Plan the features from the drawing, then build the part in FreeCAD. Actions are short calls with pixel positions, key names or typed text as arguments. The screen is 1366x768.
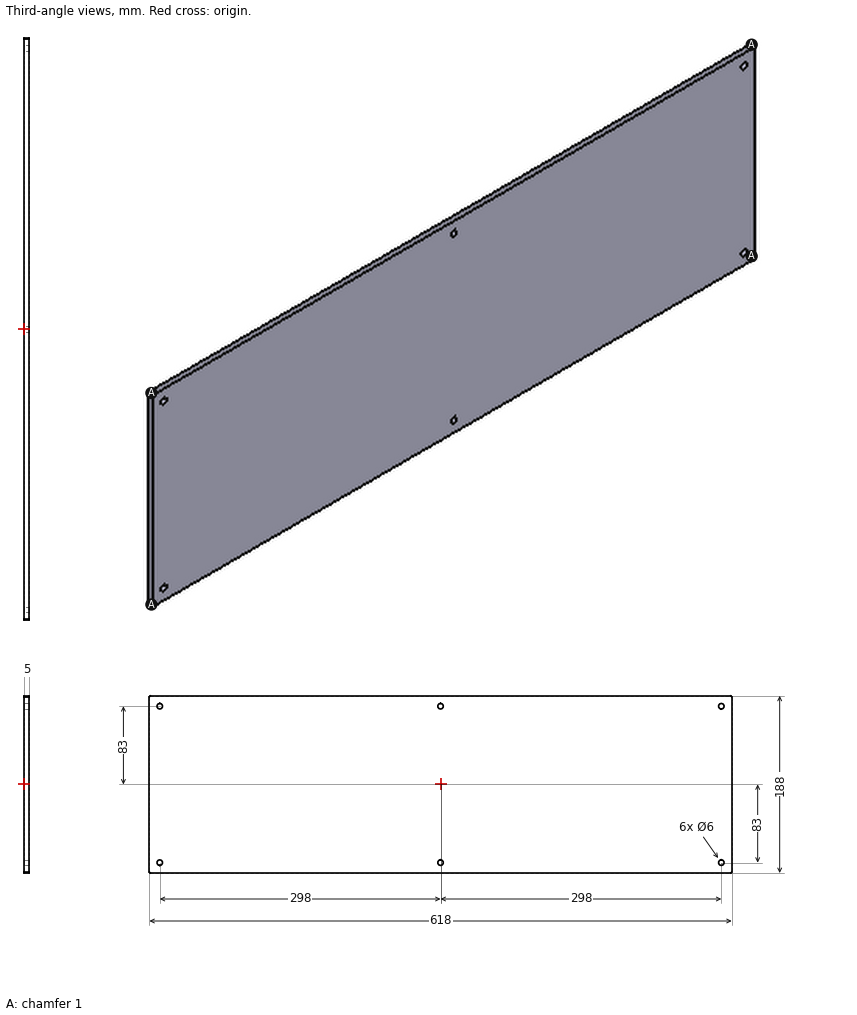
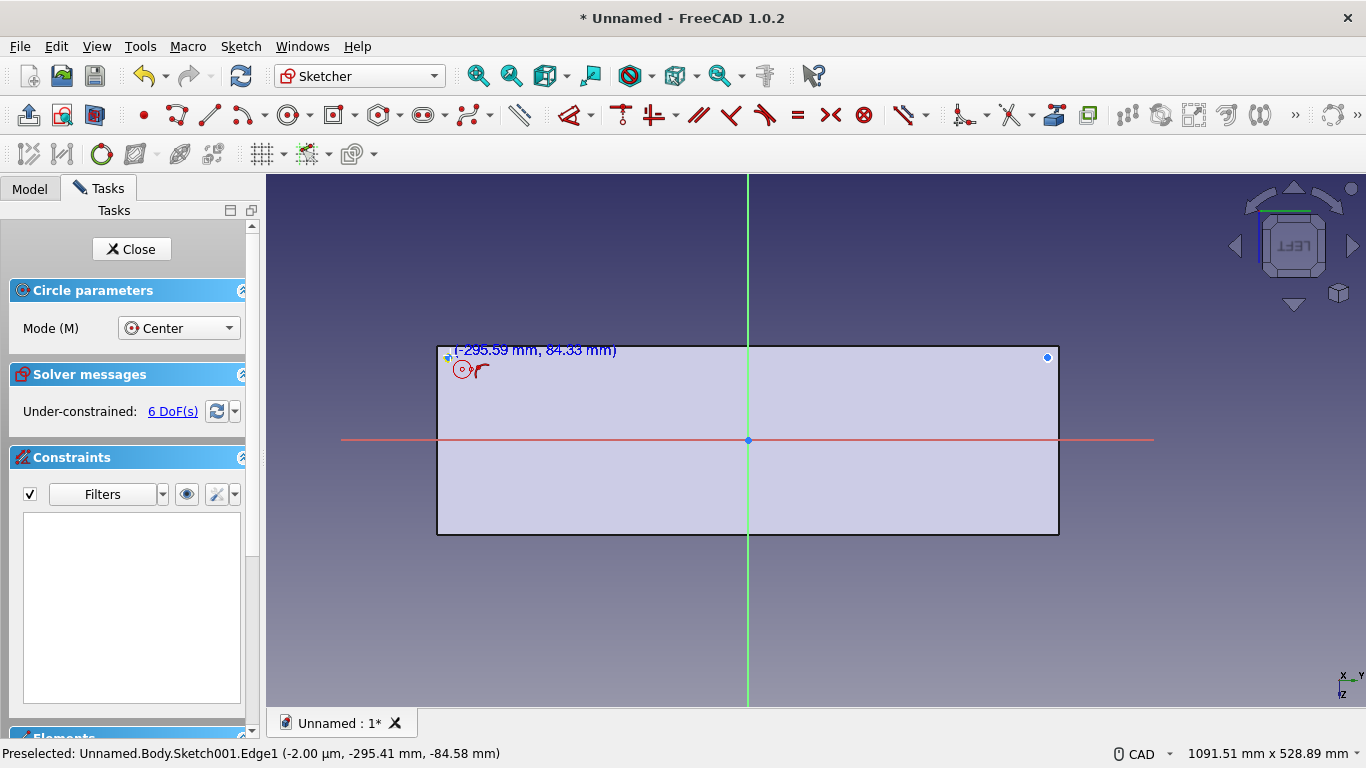
scroll(448, 524, up, 11)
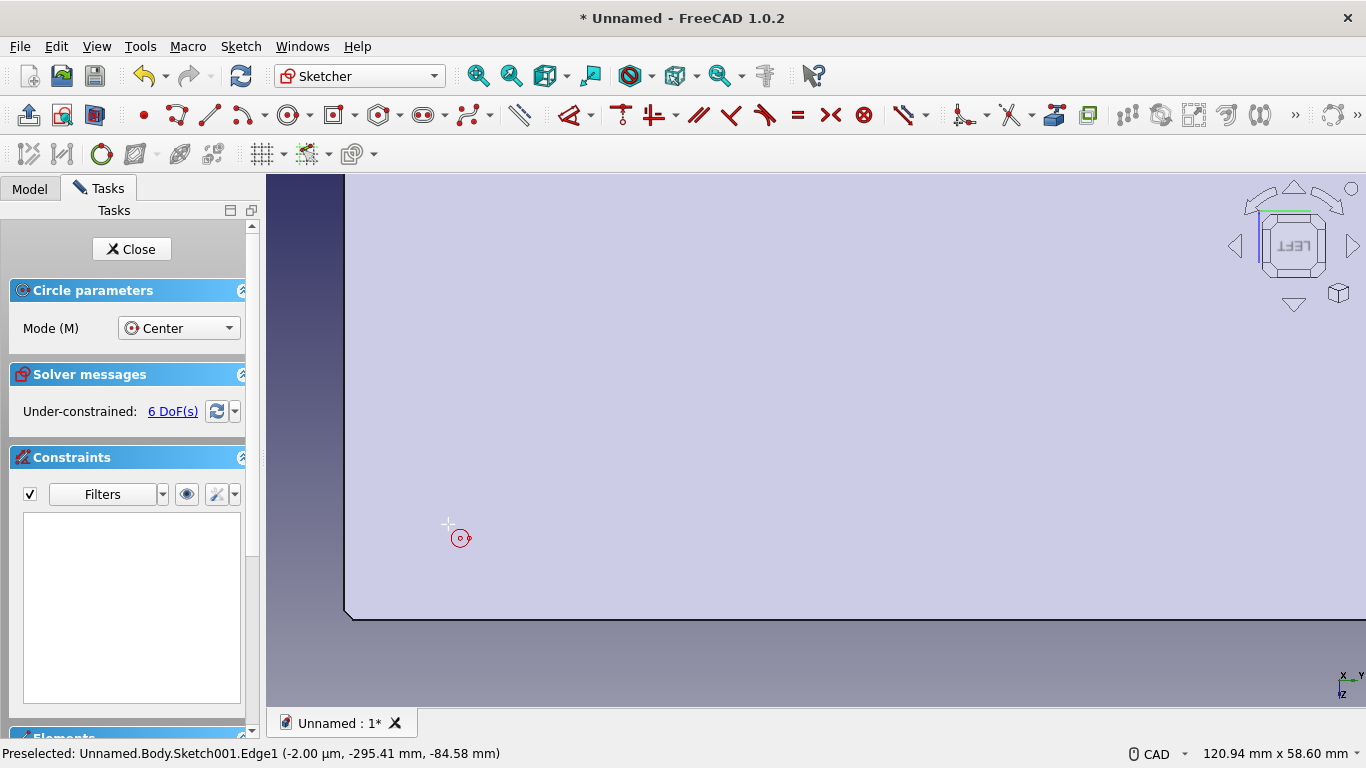
scroll(448, 525, down, 11)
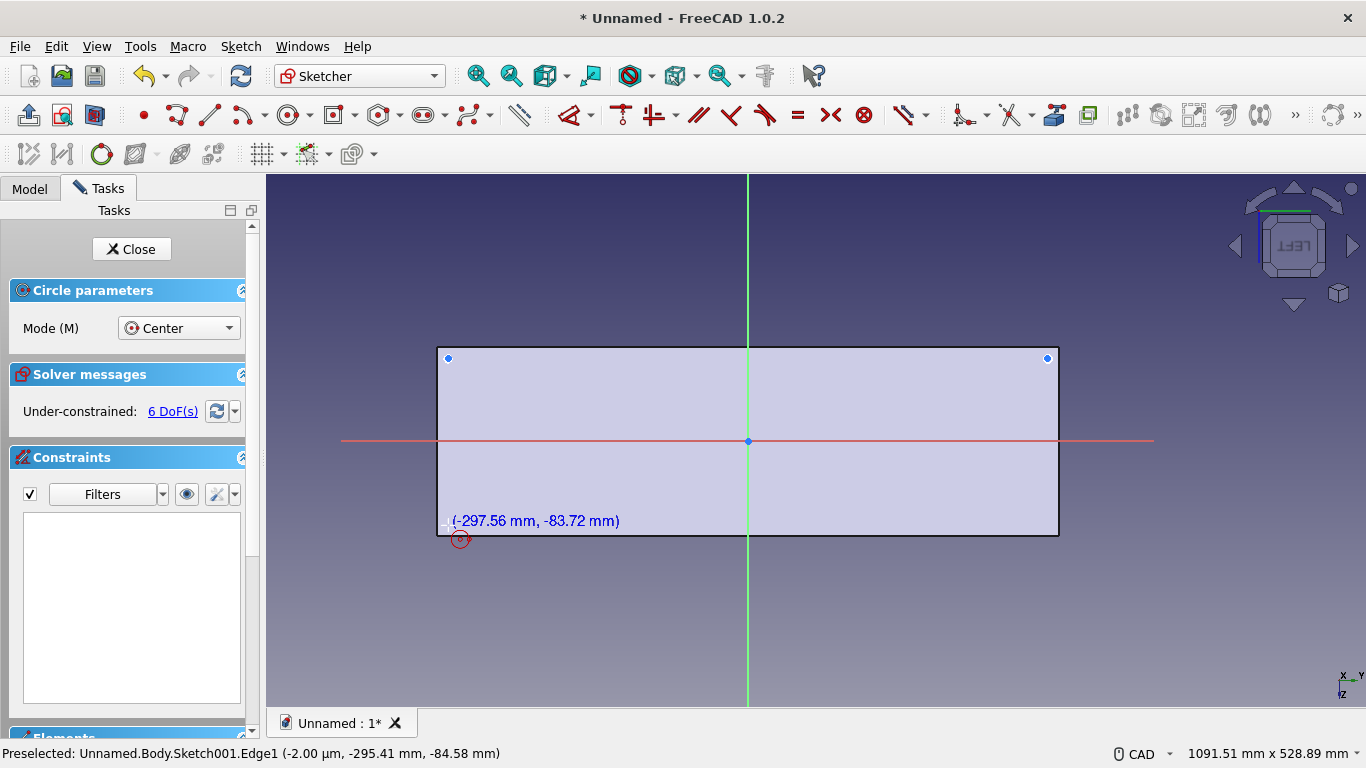
click(448, 525)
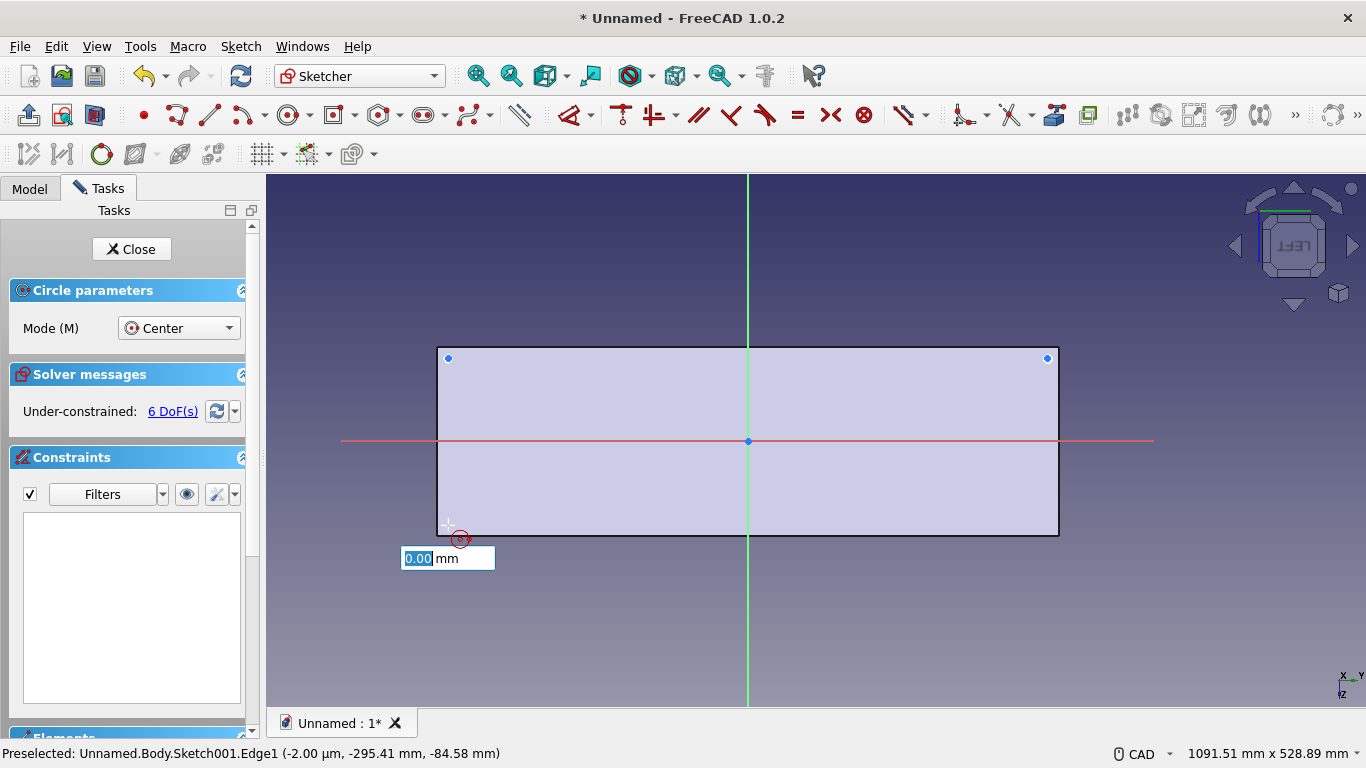
scroll(450, 523, up, 9)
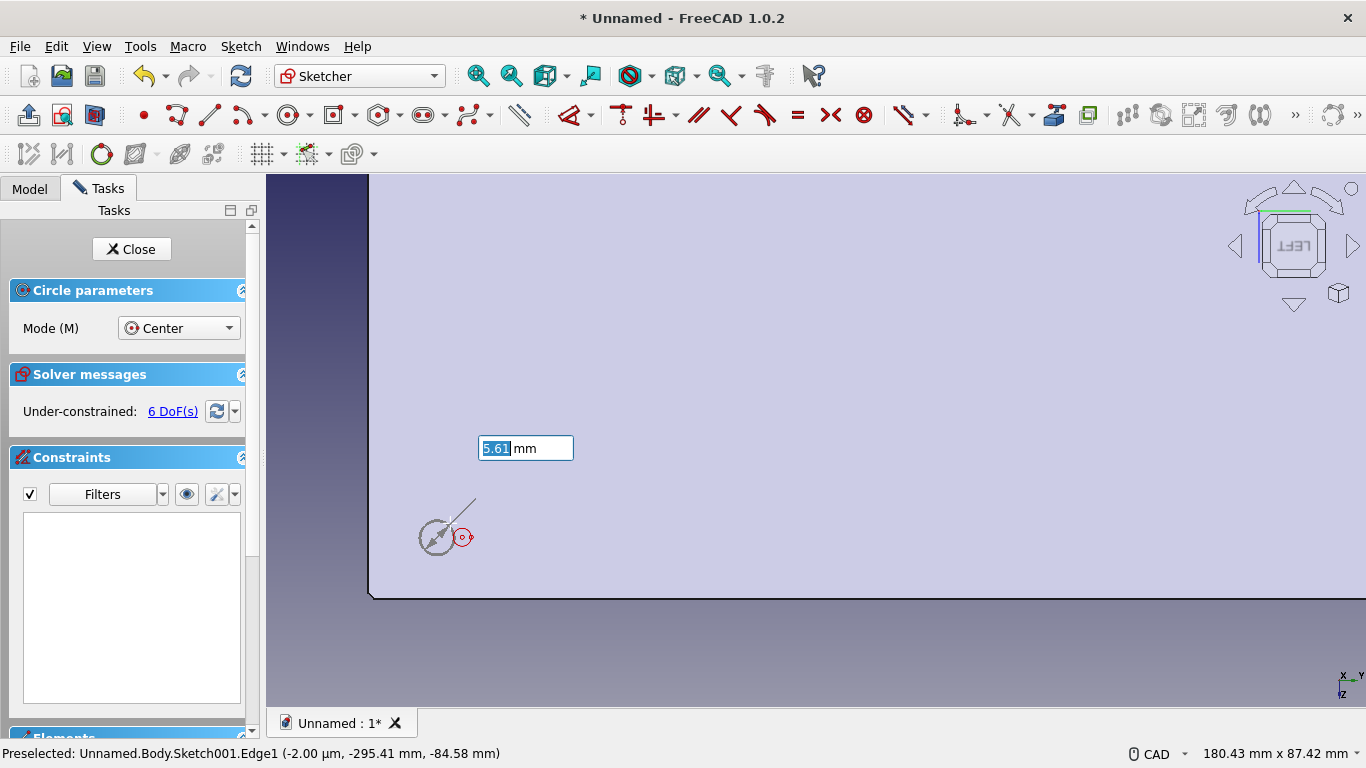
click(448, 519)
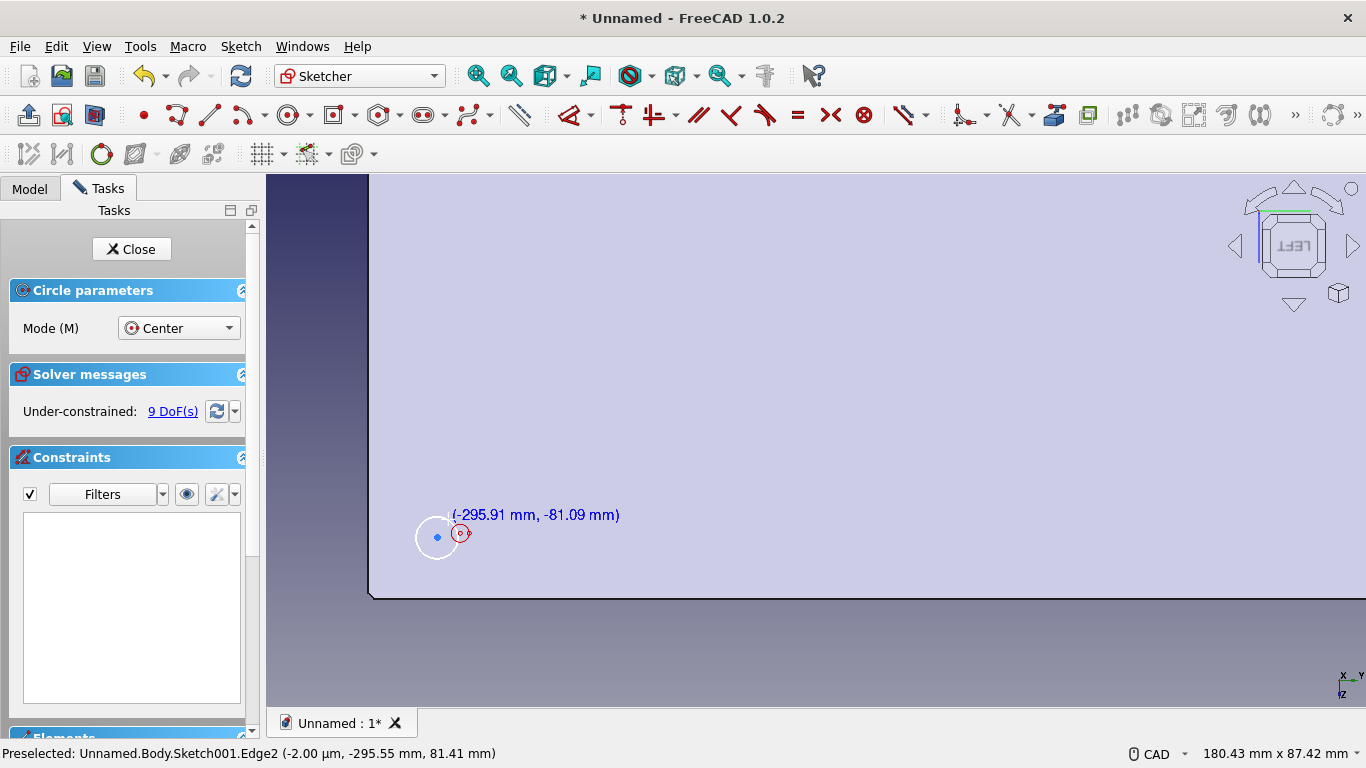
scroll(450, 523, down, 9)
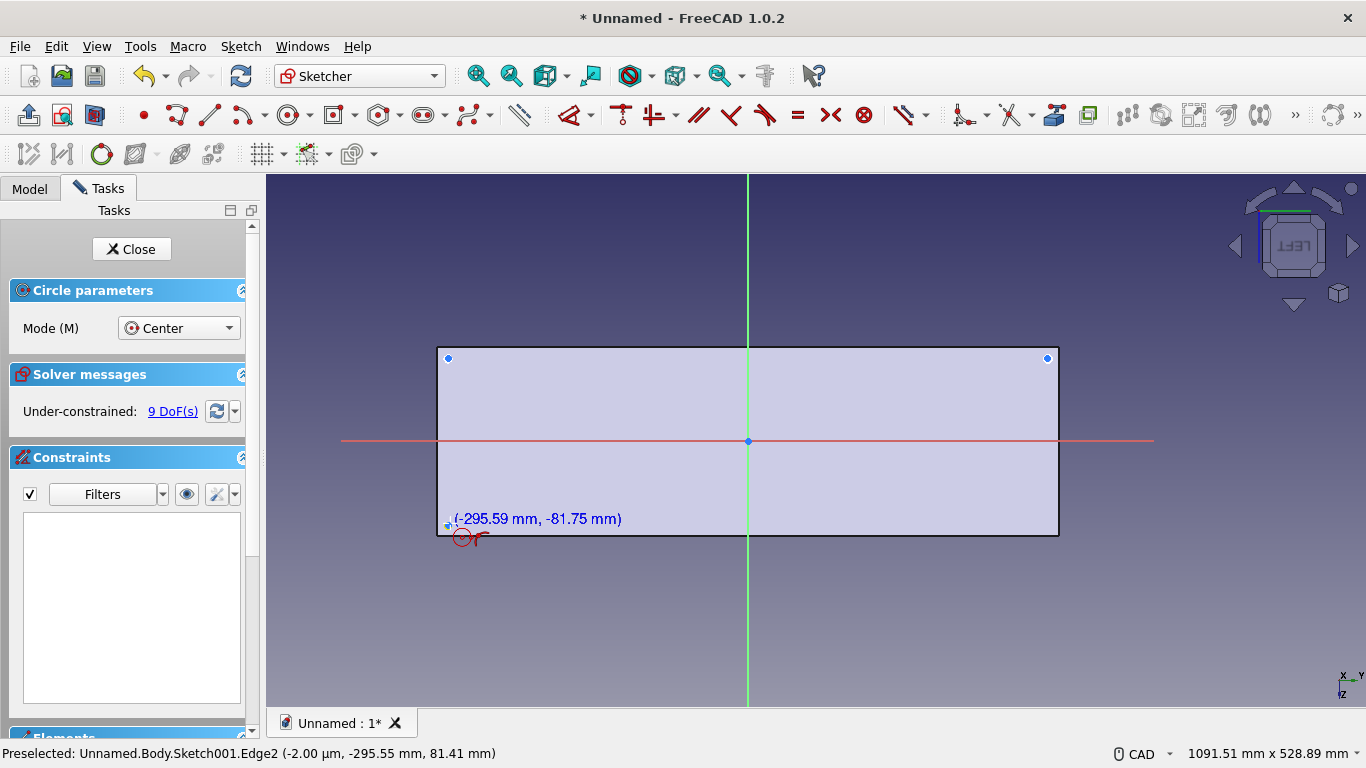
scroll(1048, 525, up, 11)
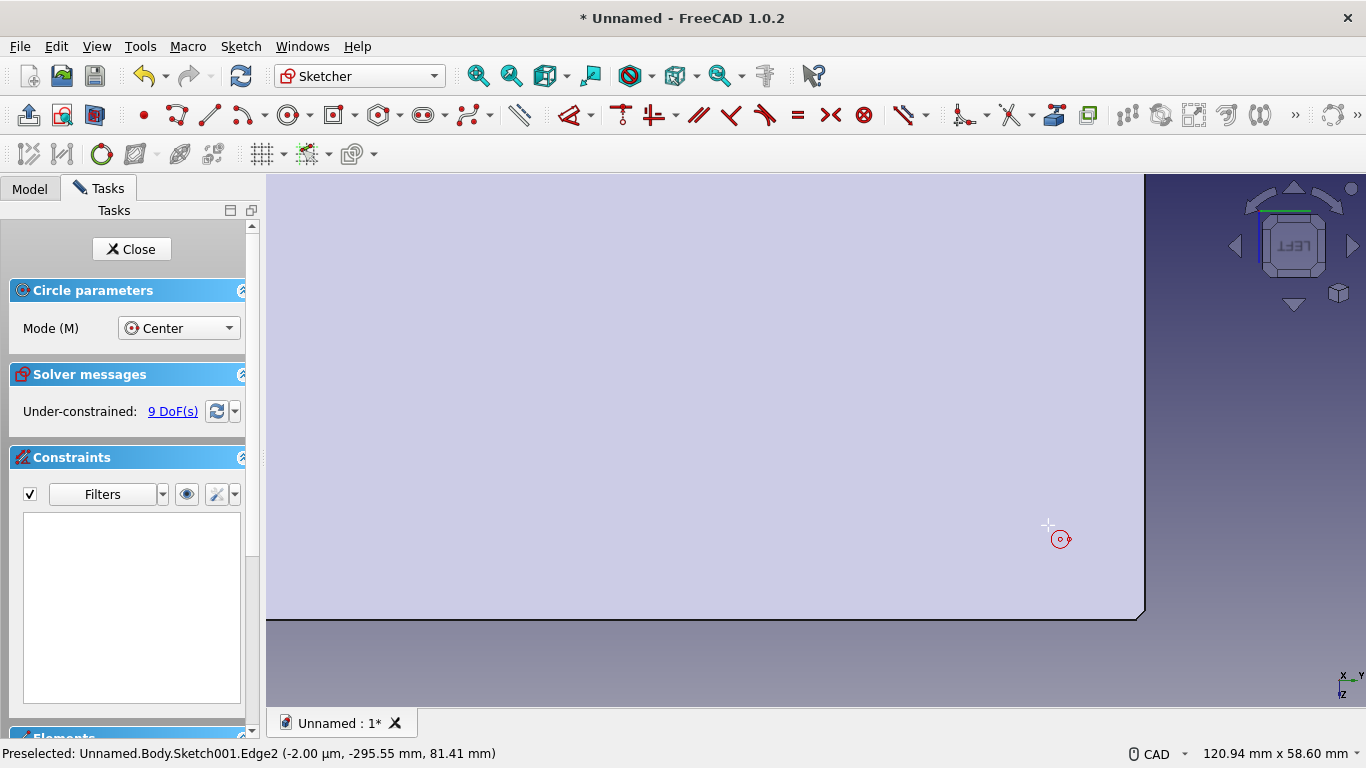
scroll(1048, 525, down, 11)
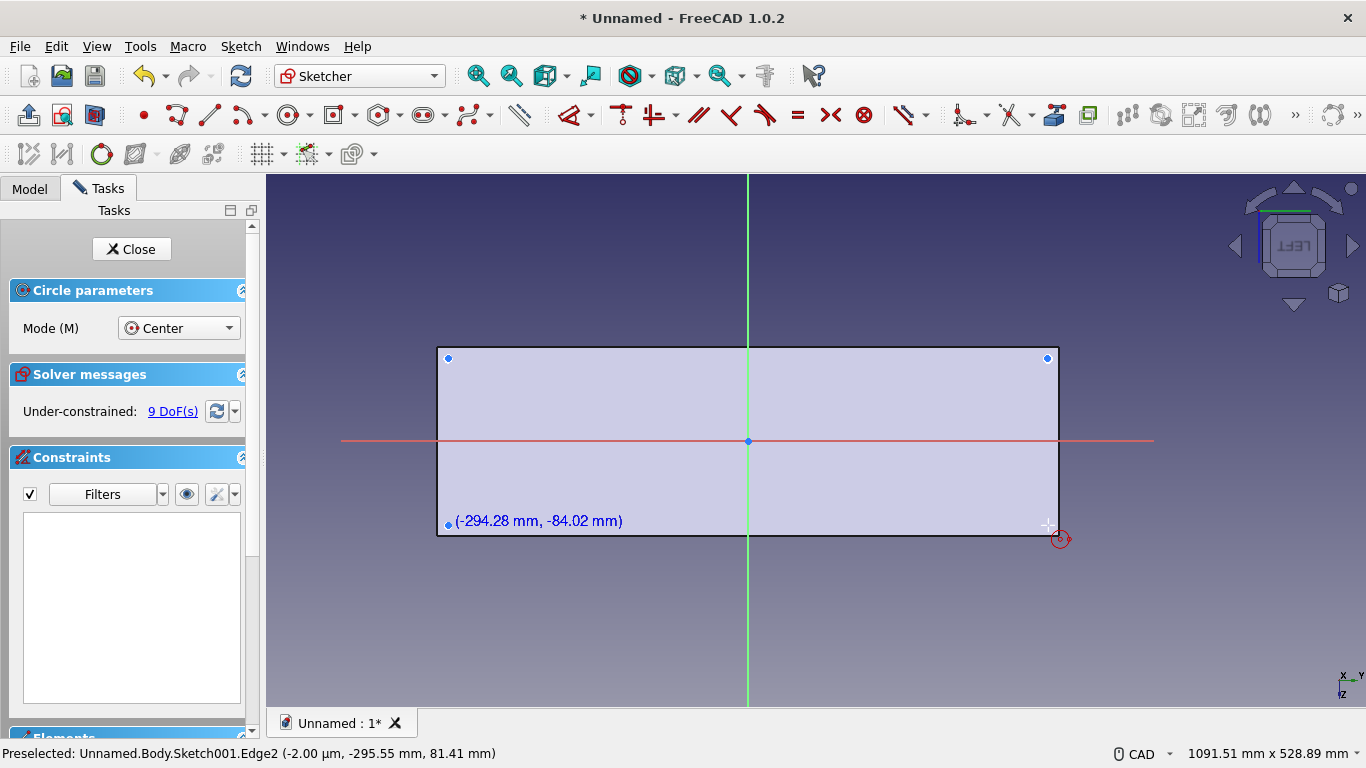
click(1048, 525)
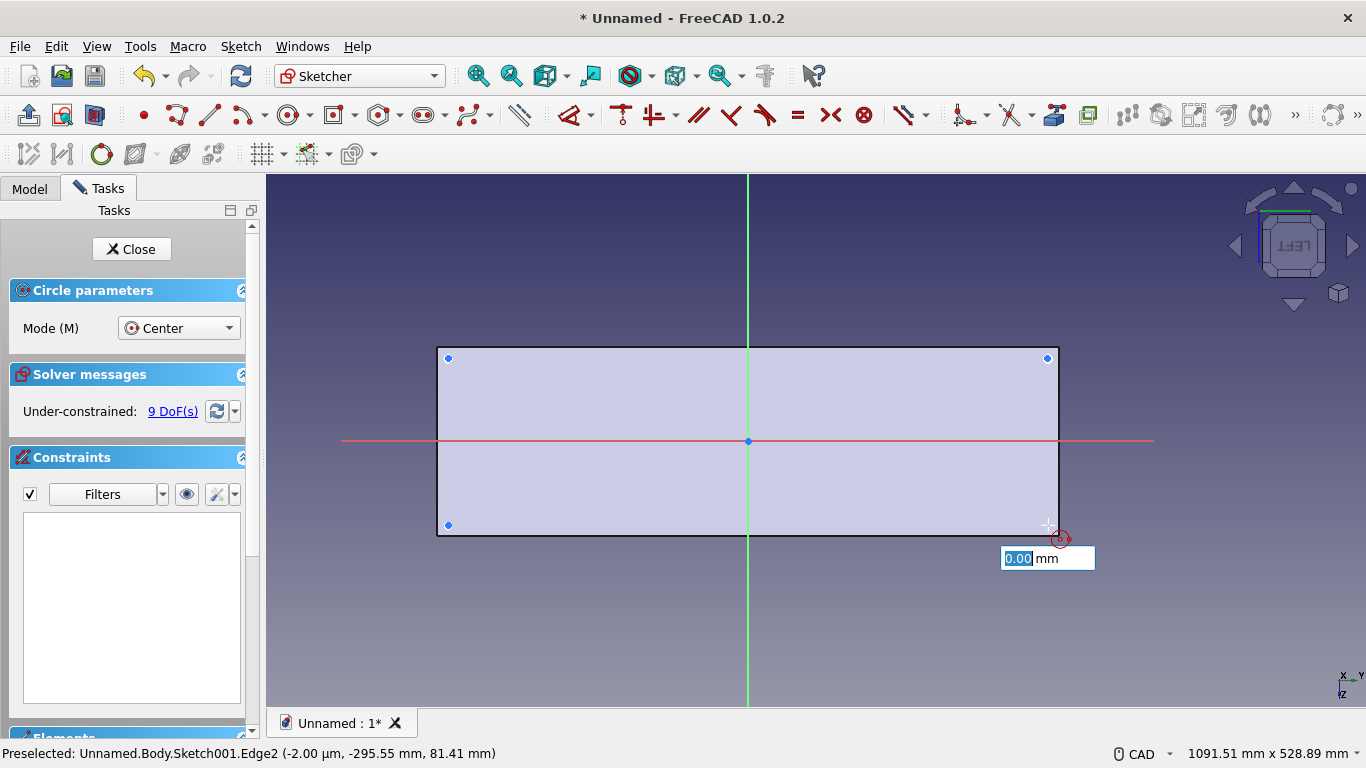
scroll(1050, 523, up, 9)